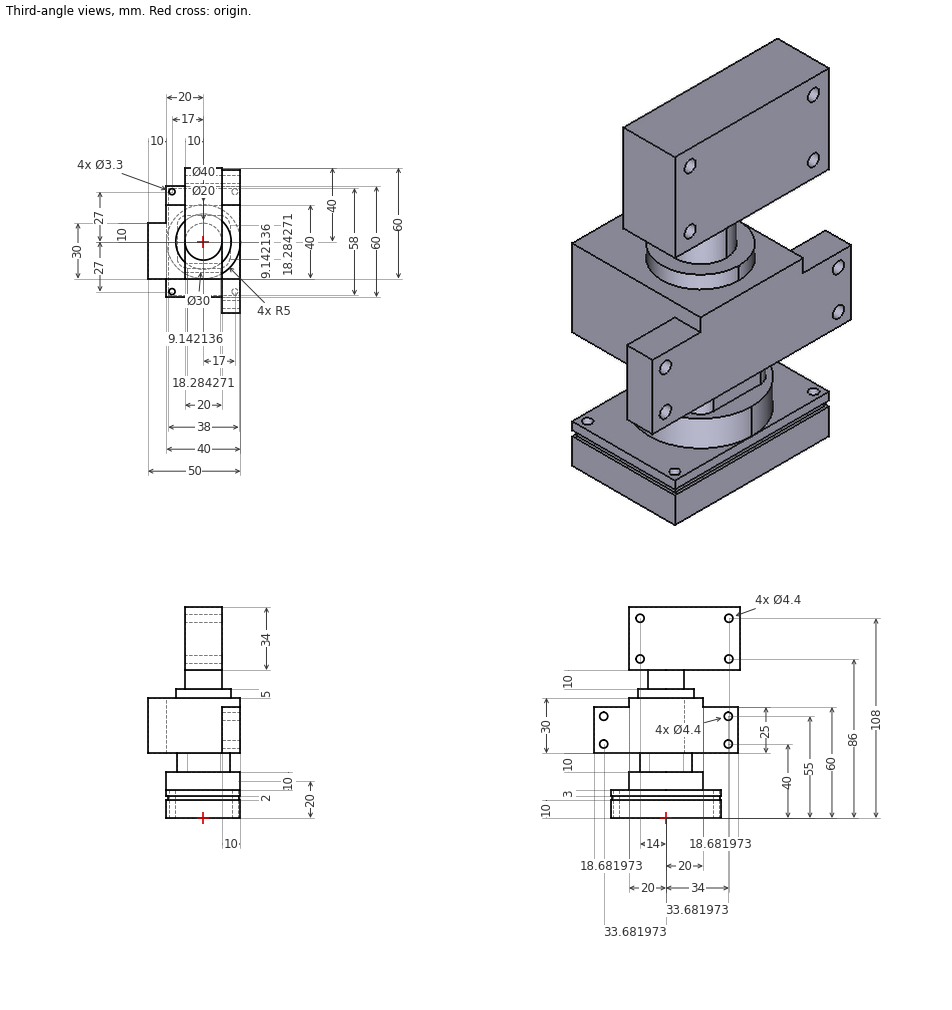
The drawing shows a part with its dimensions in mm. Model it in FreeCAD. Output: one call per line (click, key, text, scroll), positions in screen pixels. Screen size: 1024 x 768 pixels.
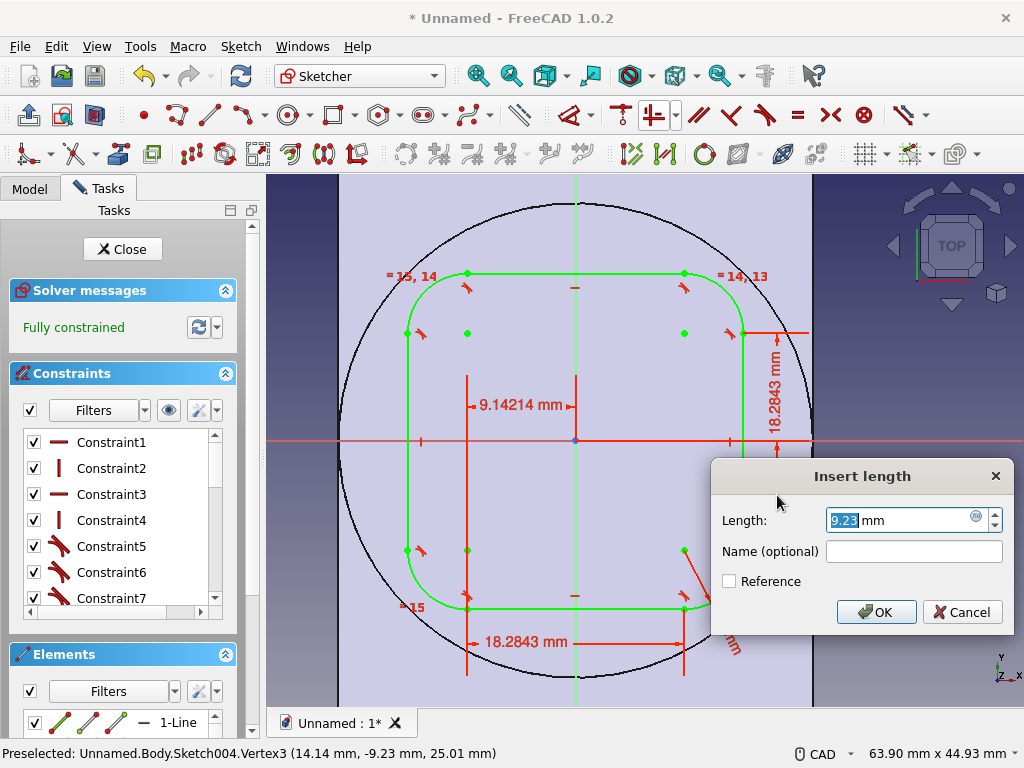
text(9.142136)
key(Return)
key(Escape)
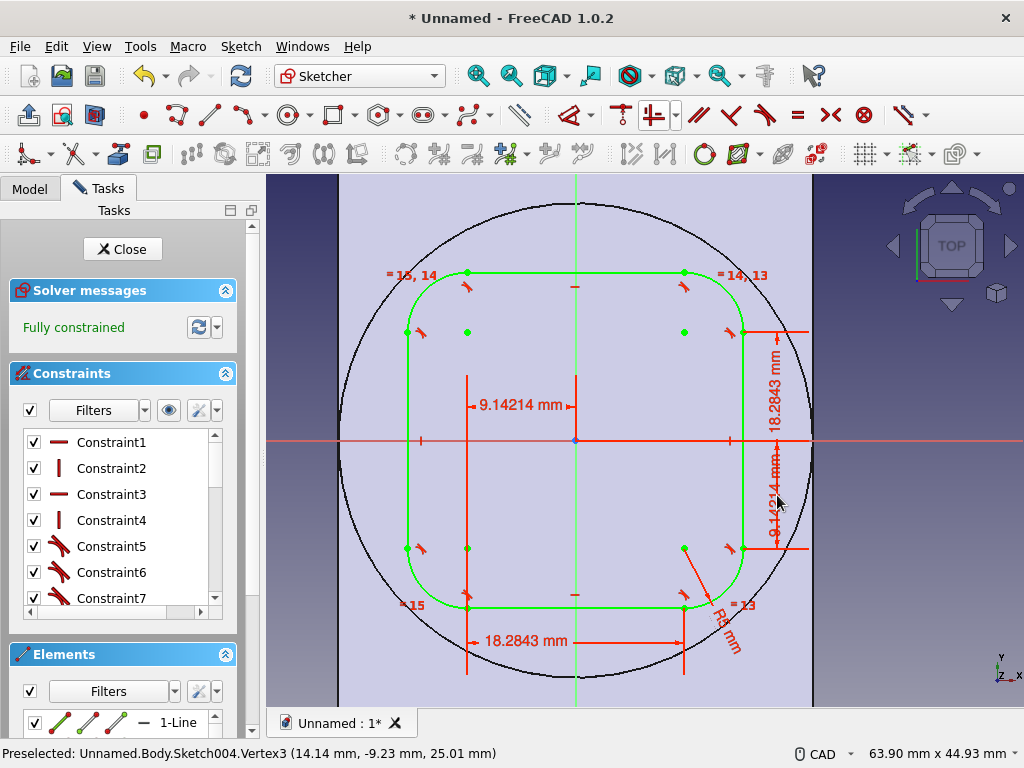
click(123, 249)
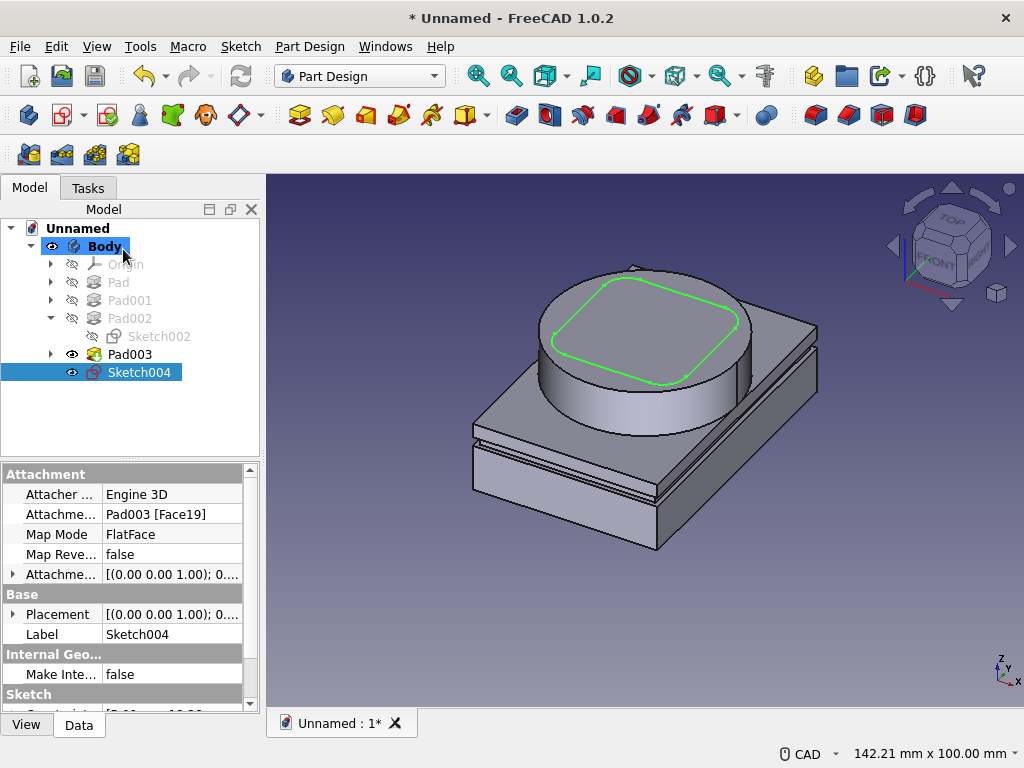
click(300, 116)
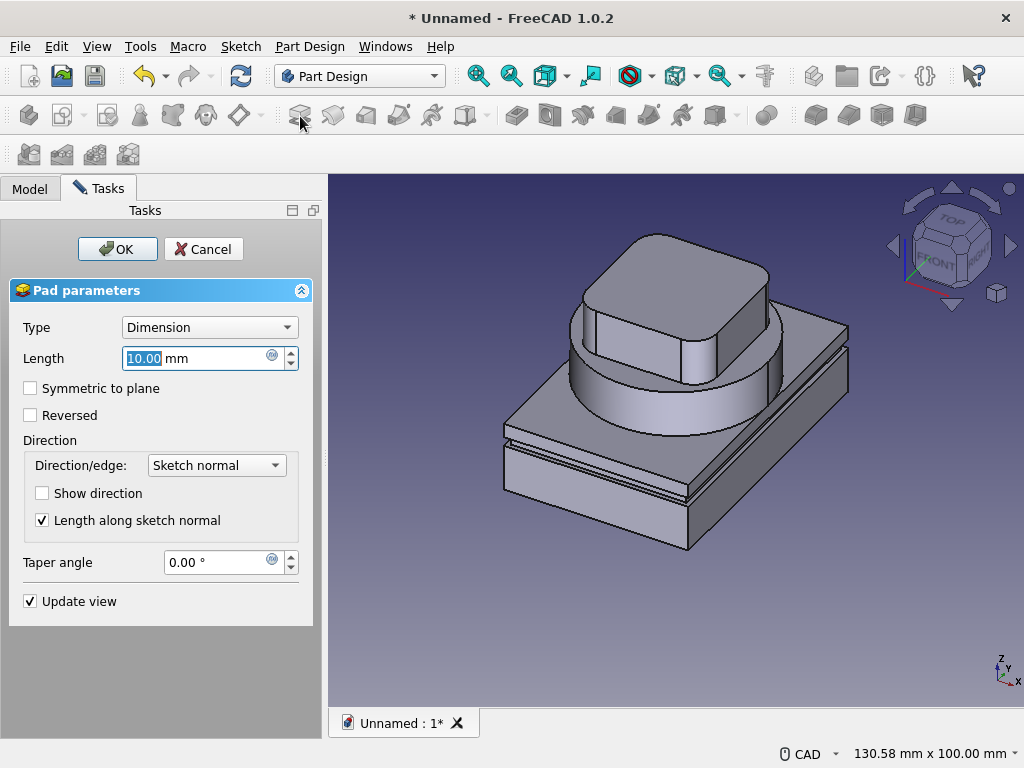
text(10)
key(Tab)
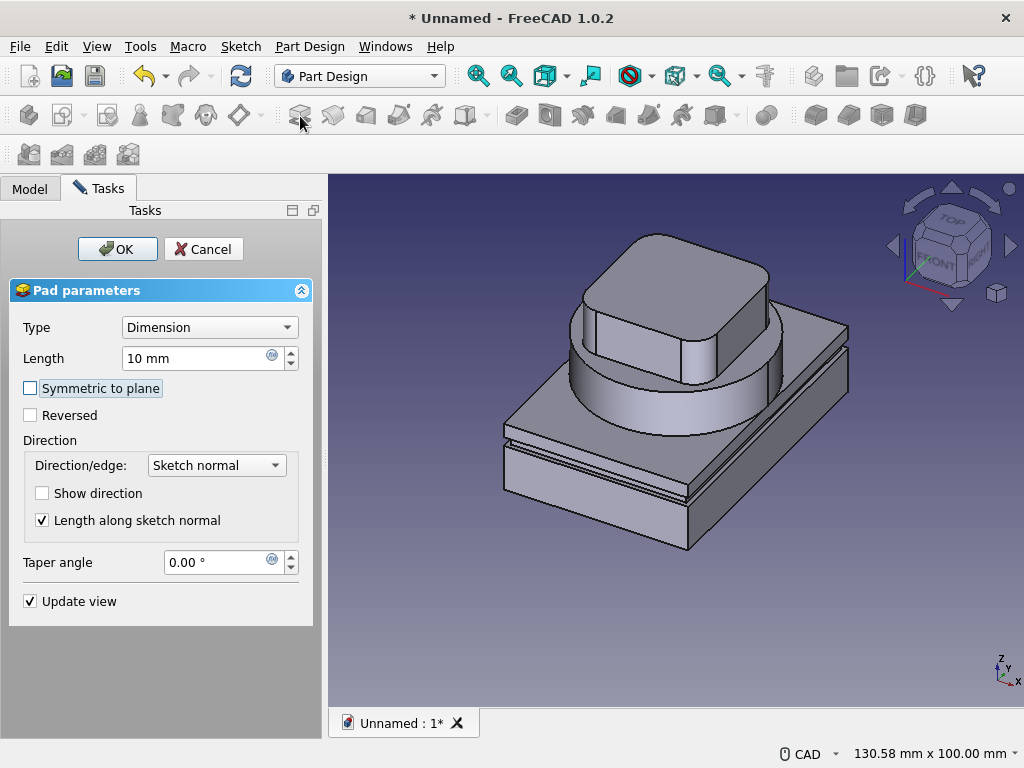
click(118, 249)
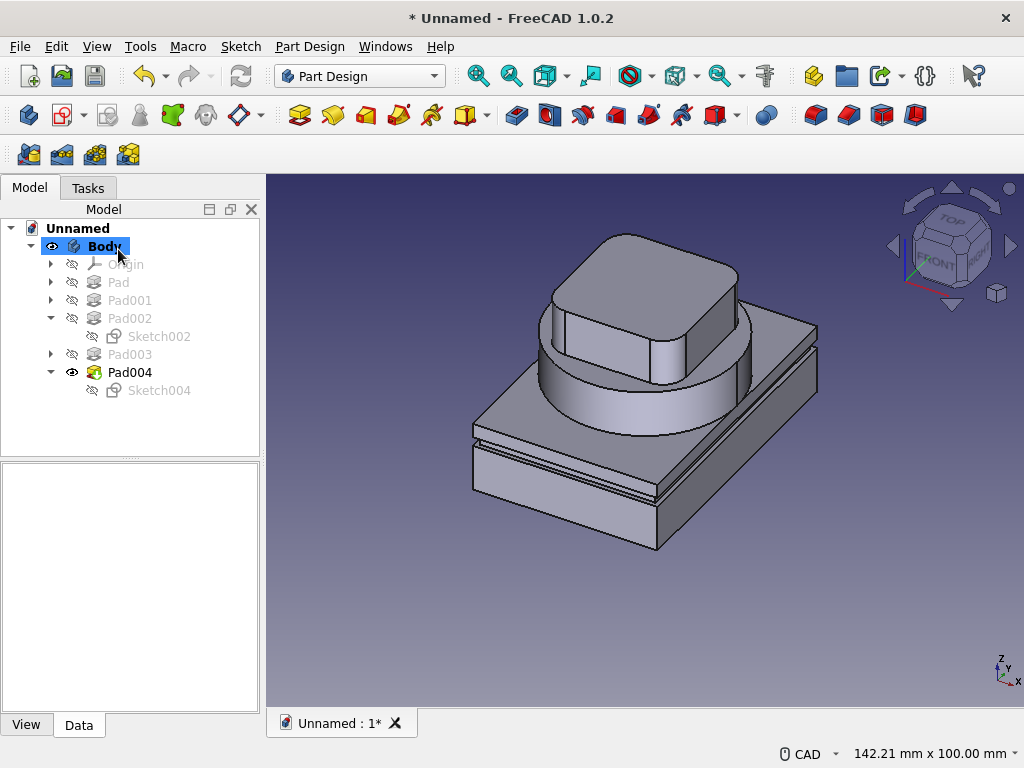
key(5)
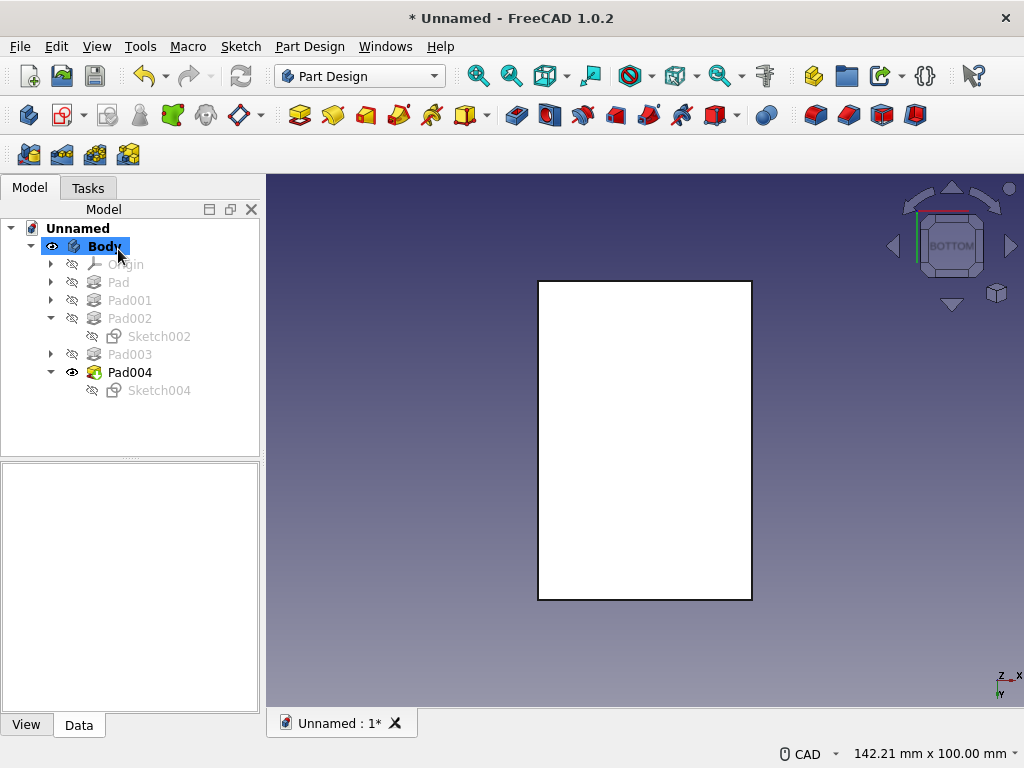
click(645, 485)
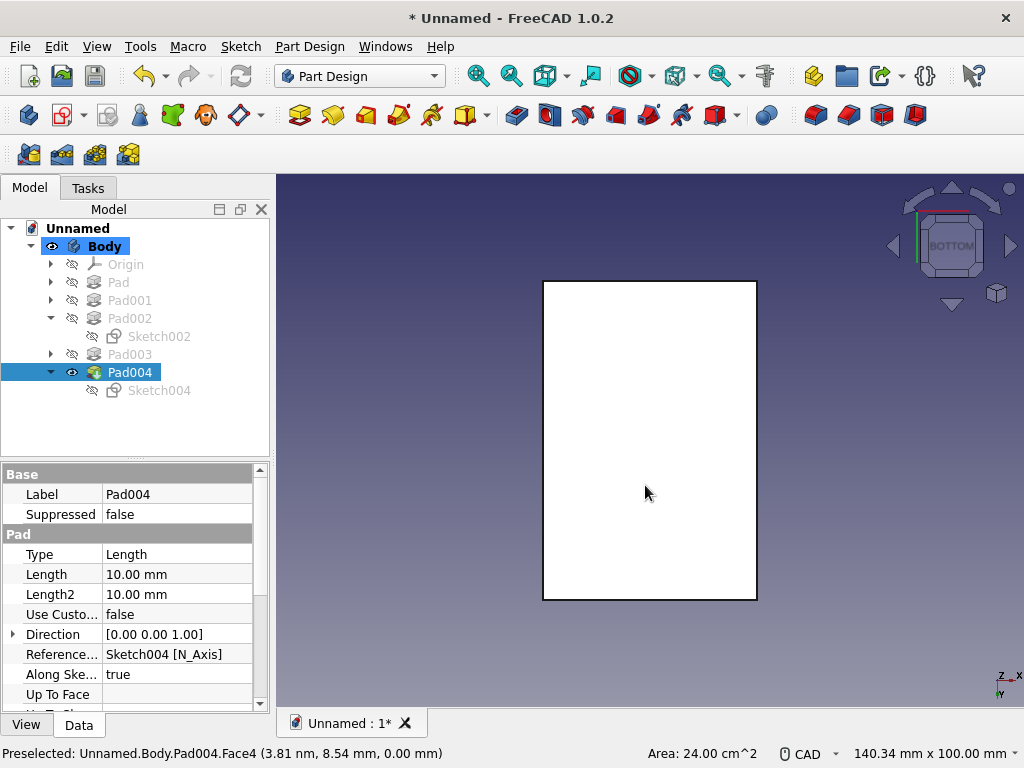
click(62, 116)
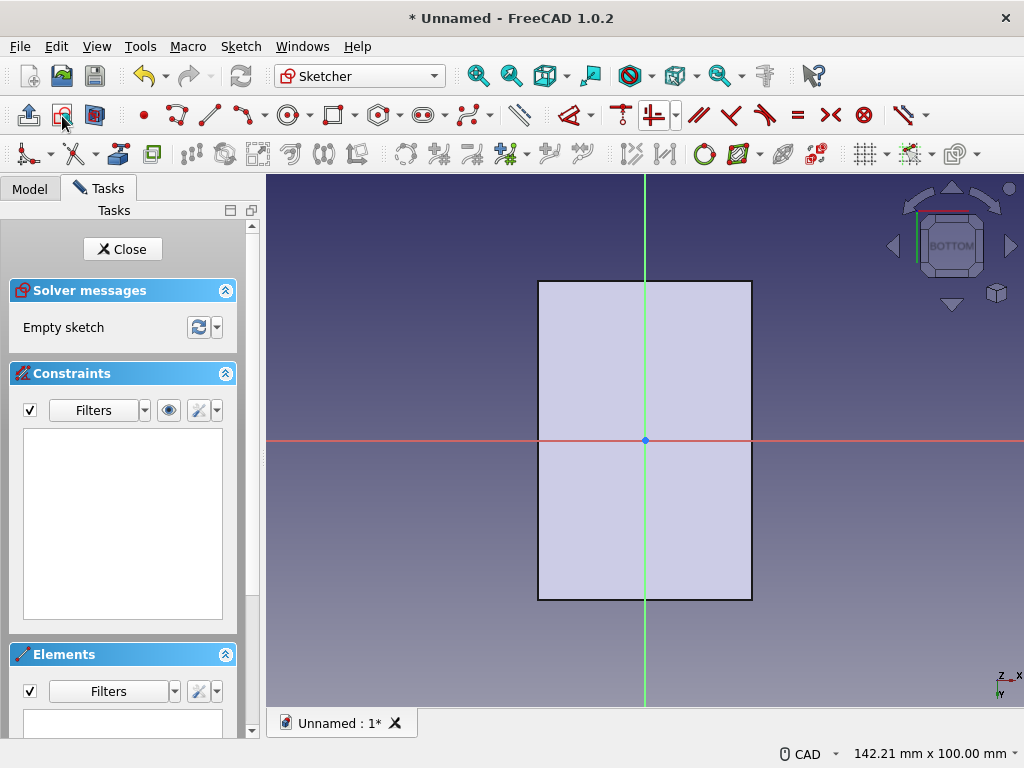
key(g)
key(c)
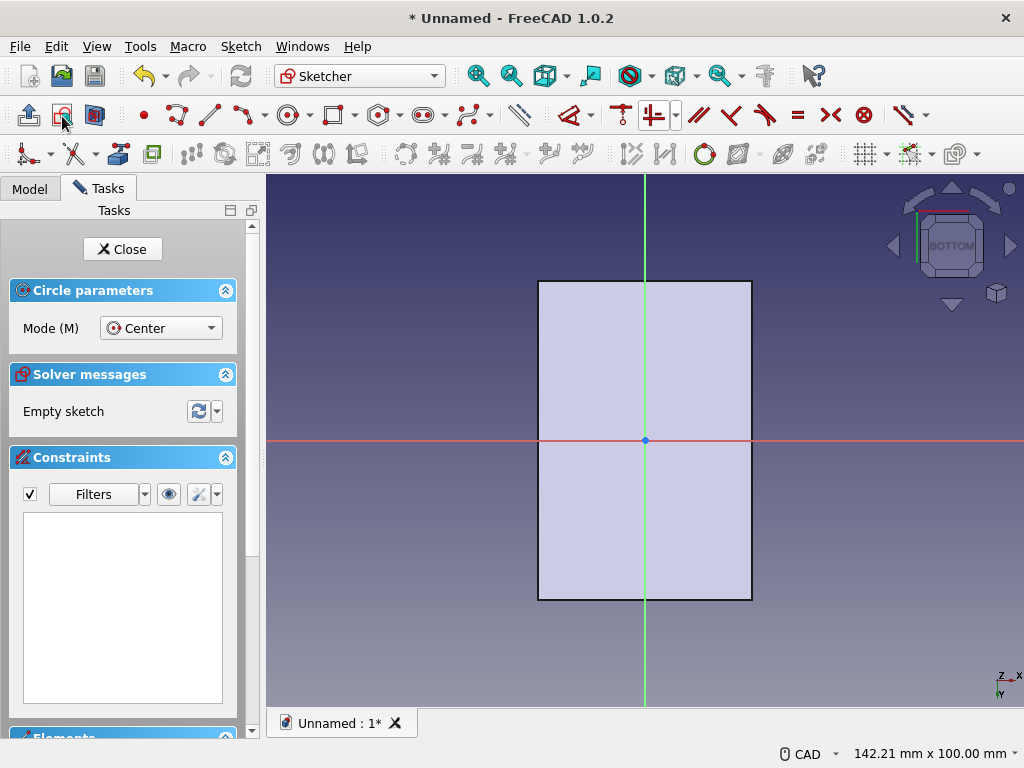
scroll(554, 584, up, 5)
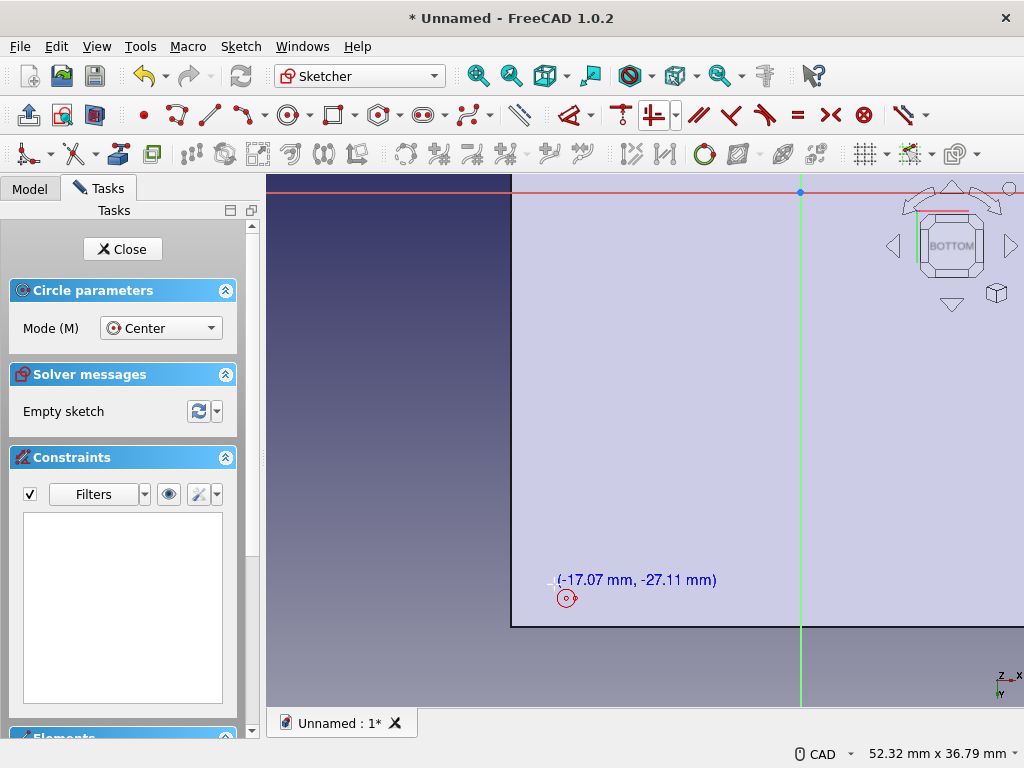
click(554, 584)
move(571, 567)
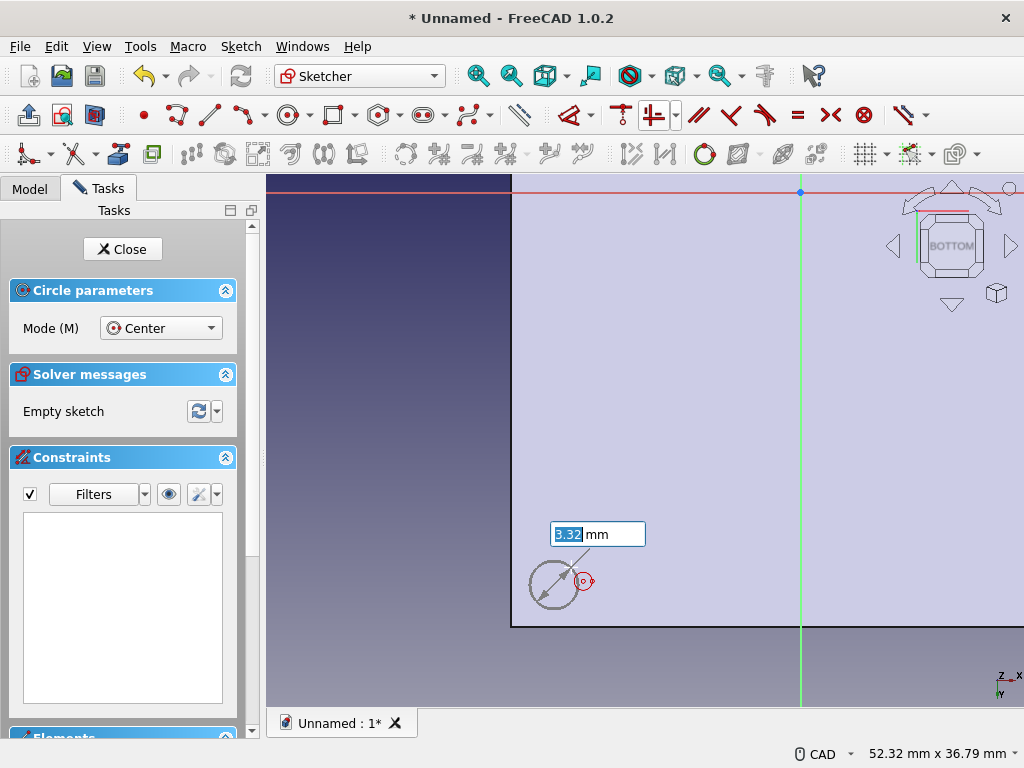
text(3.3)
key(Return)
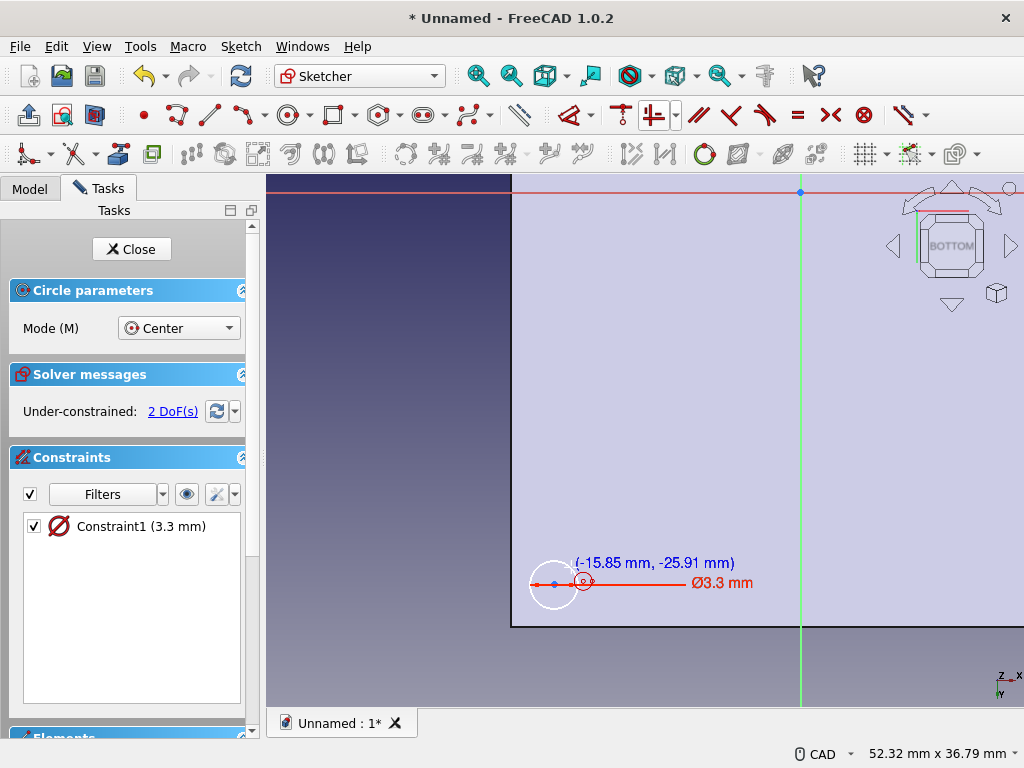
scroll(446, 585, down, 5)